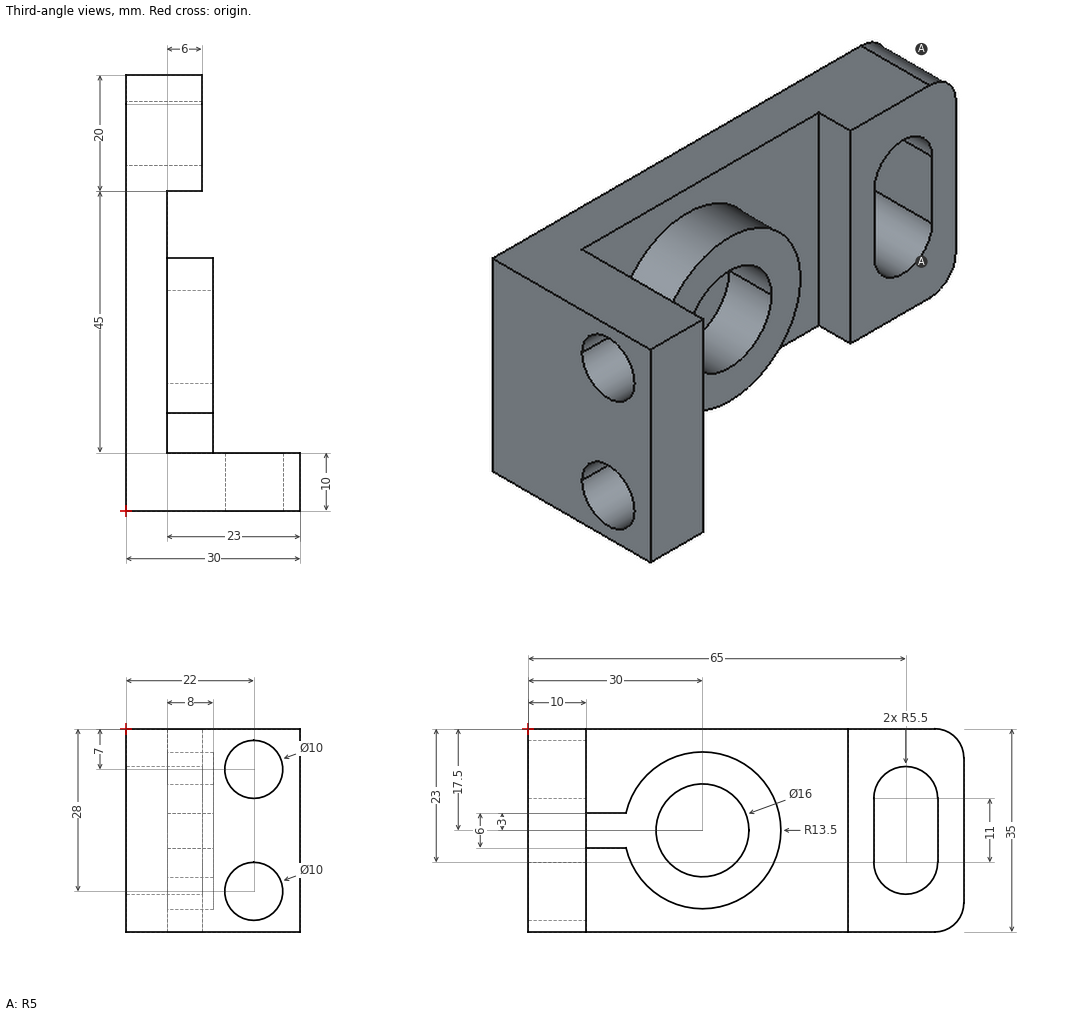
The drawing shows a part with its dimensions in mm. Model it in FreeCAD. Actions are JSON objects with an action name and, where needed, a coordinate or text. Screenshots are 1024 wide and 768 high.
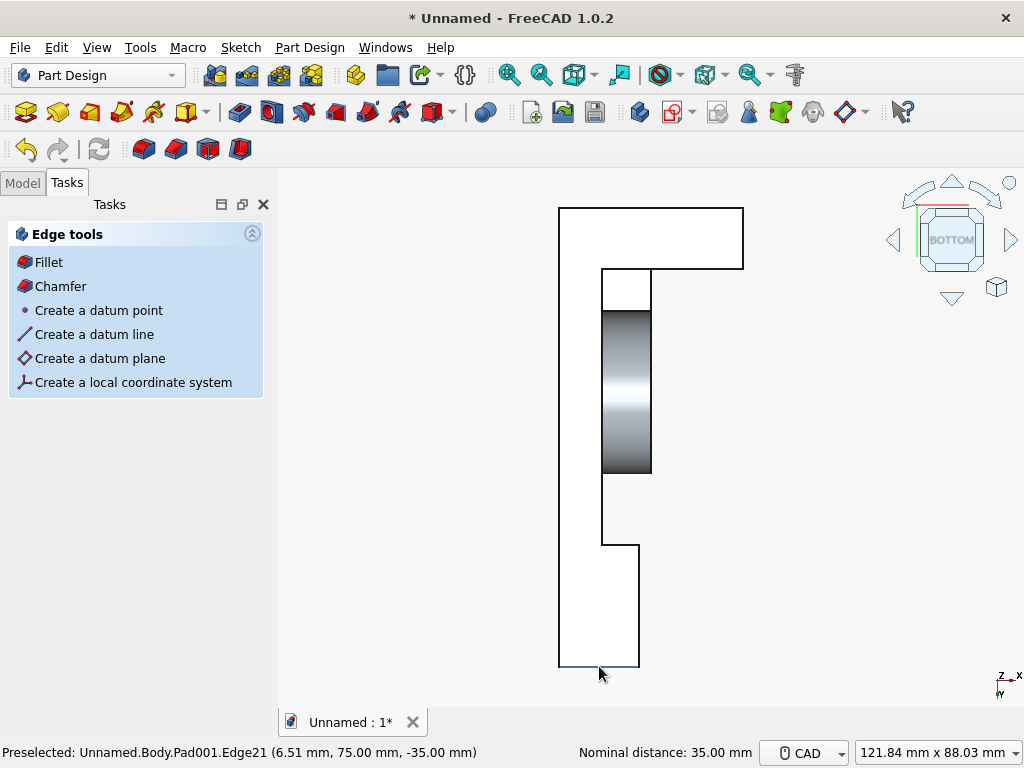
{"action": "left_click", "coordinate": [144, 150]}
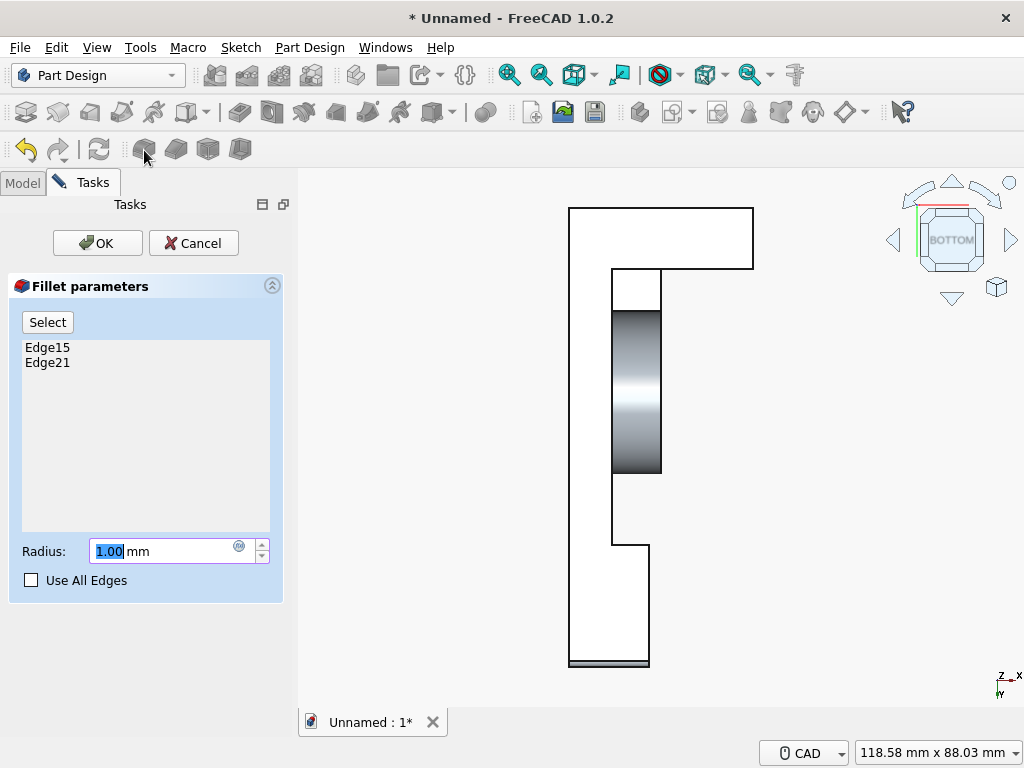
{"action": "type", "text": "5"}
{"action": "key", "text": "Tab"}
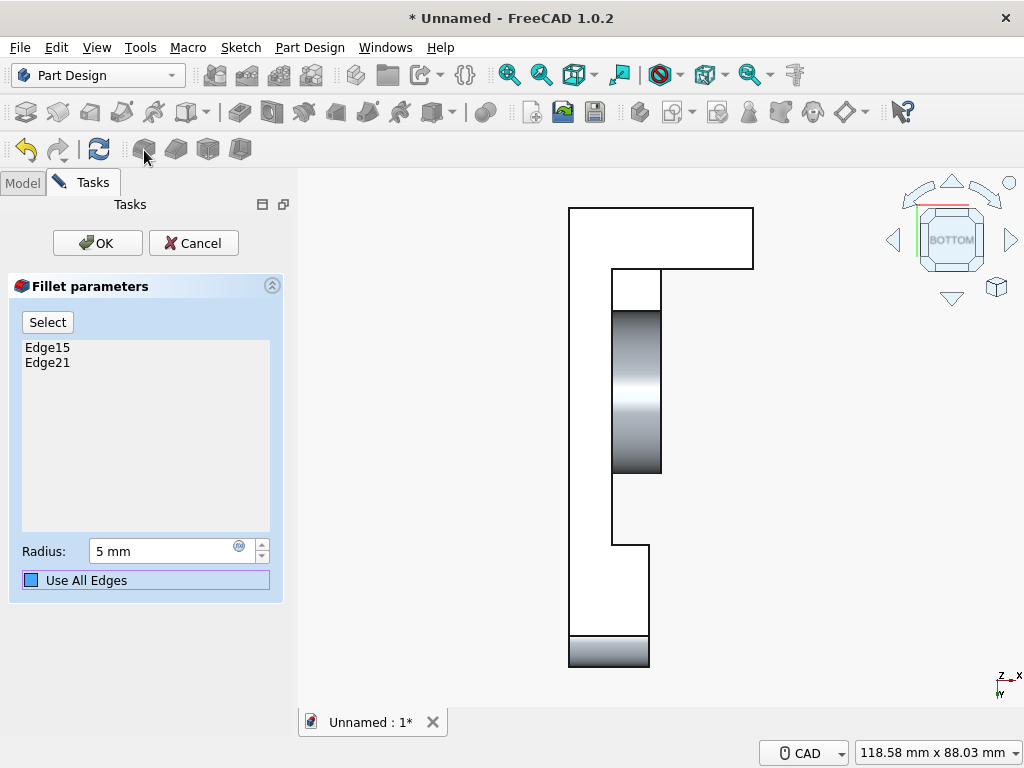
{"action": "left_click", "coordinate": [98, 243]}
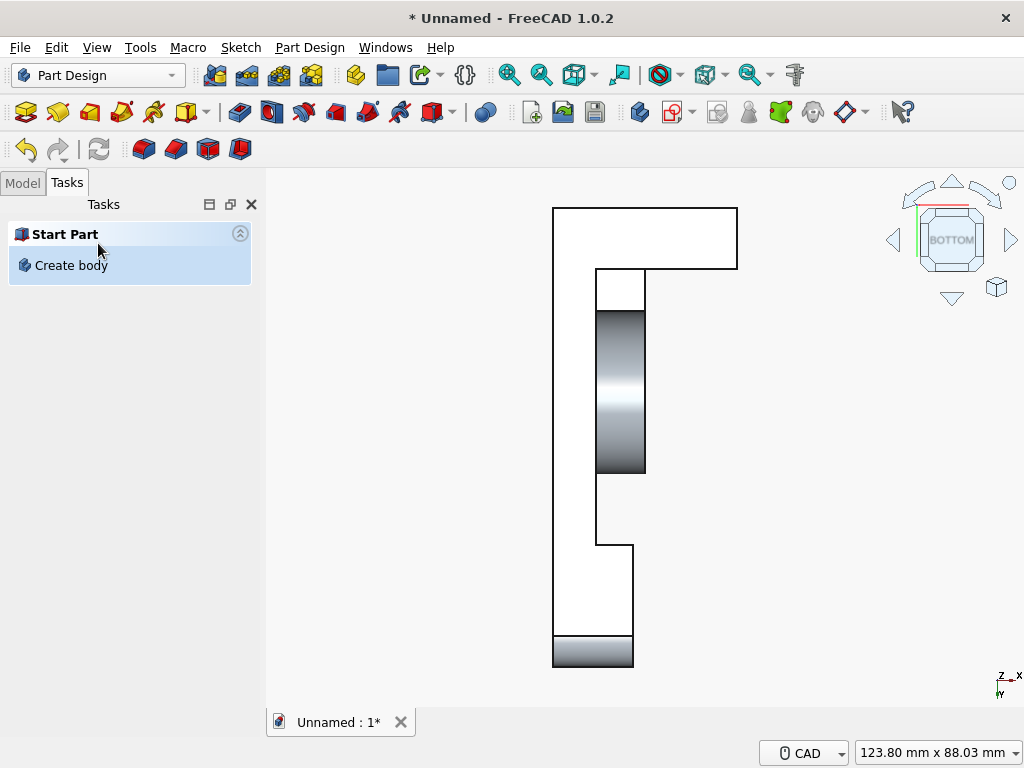
{"action": "key", "text": "0"}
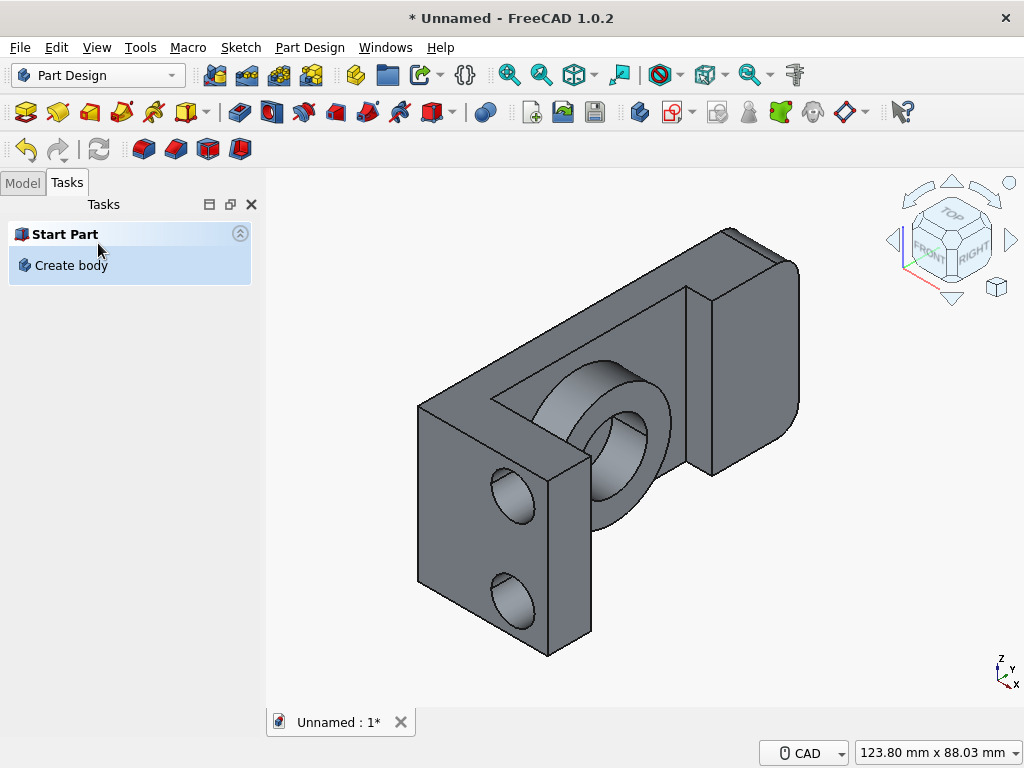
{"action": "left_click", "coordinate": [755, 338]}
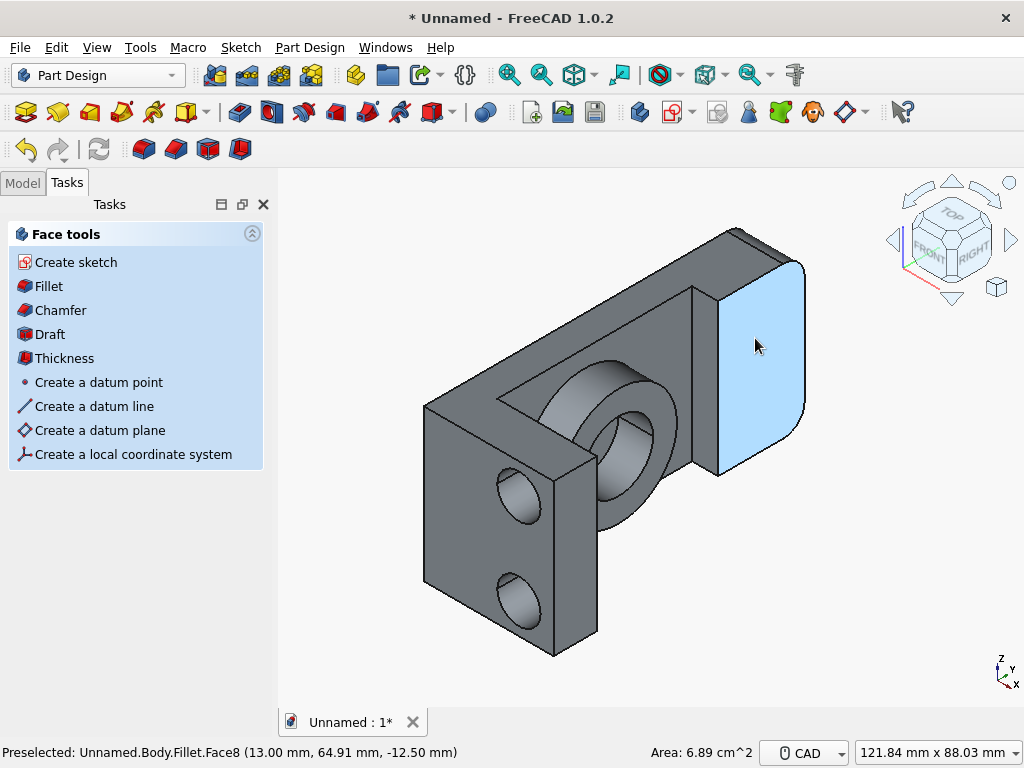
{"action": "left_click", "coordinate": [672, 112]}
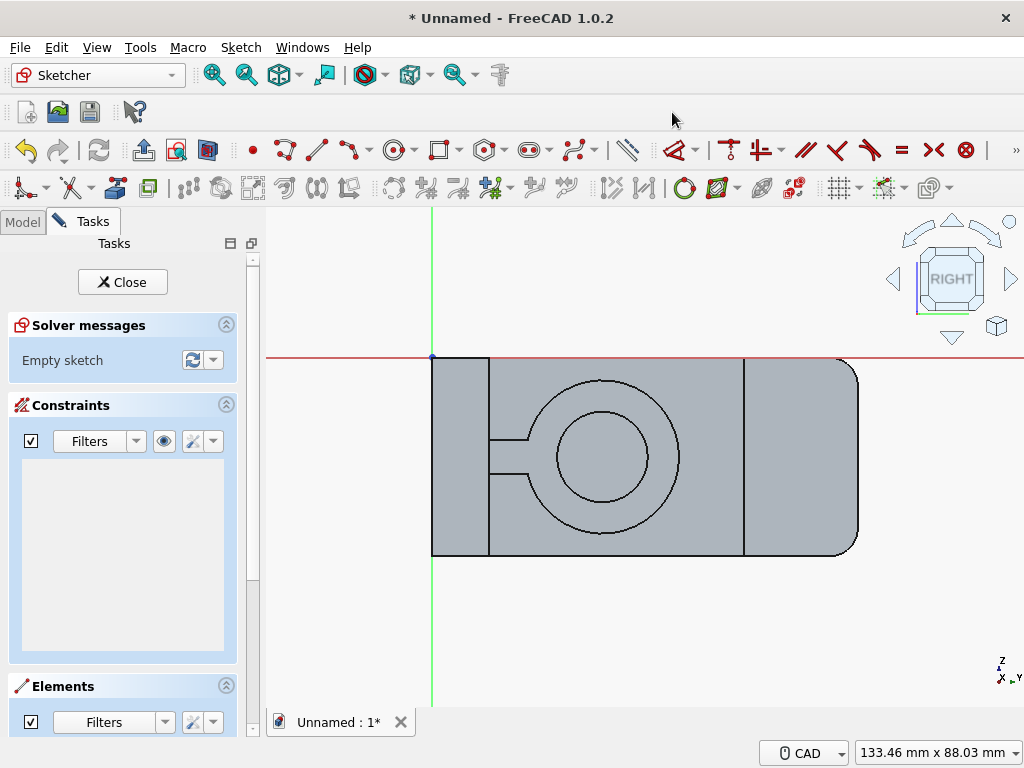
{"action": "scroll", "coordinate": [859, 457], "scroll_direction": "up", "scroll_amount": 5}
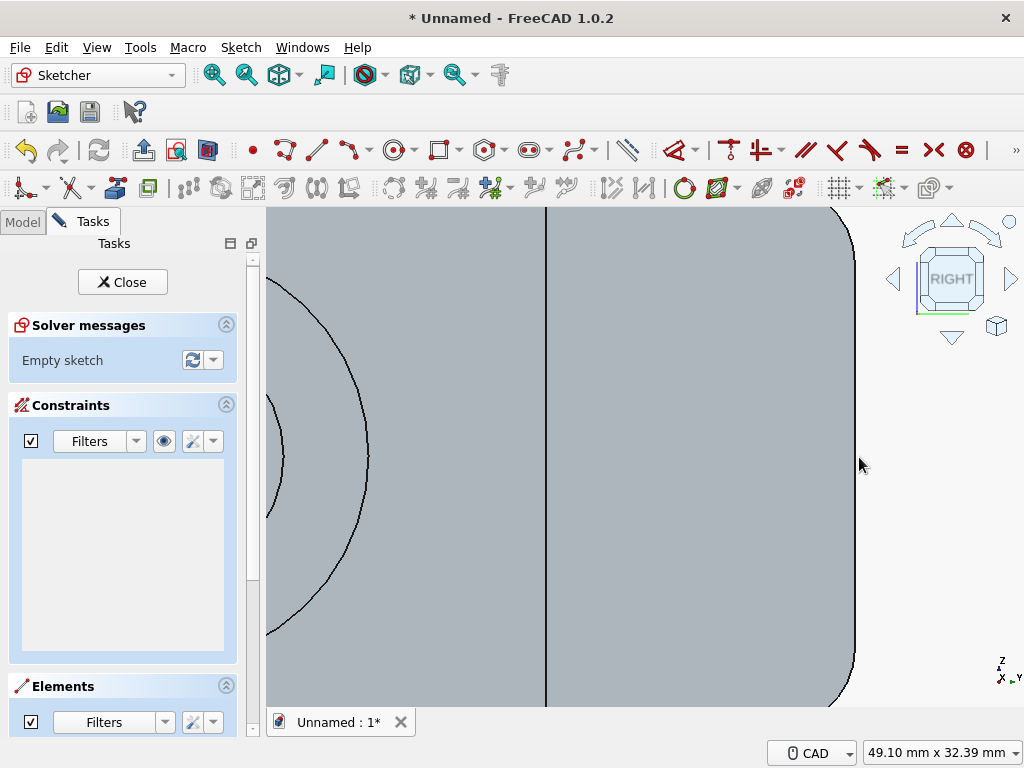
{"action": "left_click", "coordinate": [530, 150]}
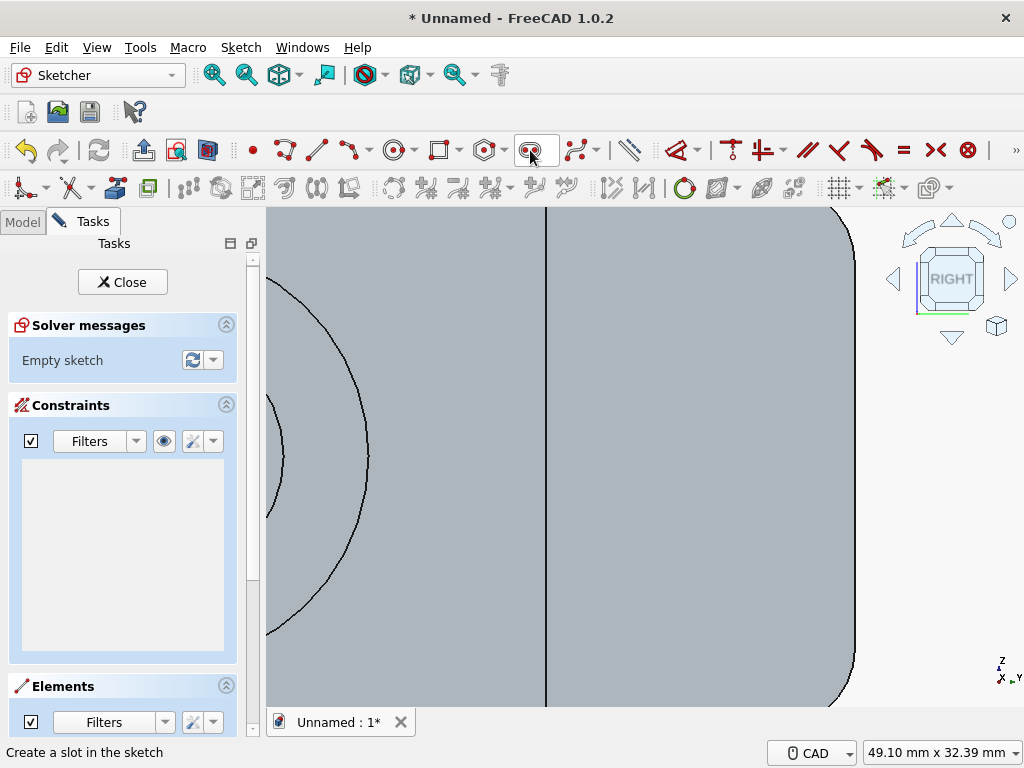
{"action": "left_click", "coordinate": [701, 541]}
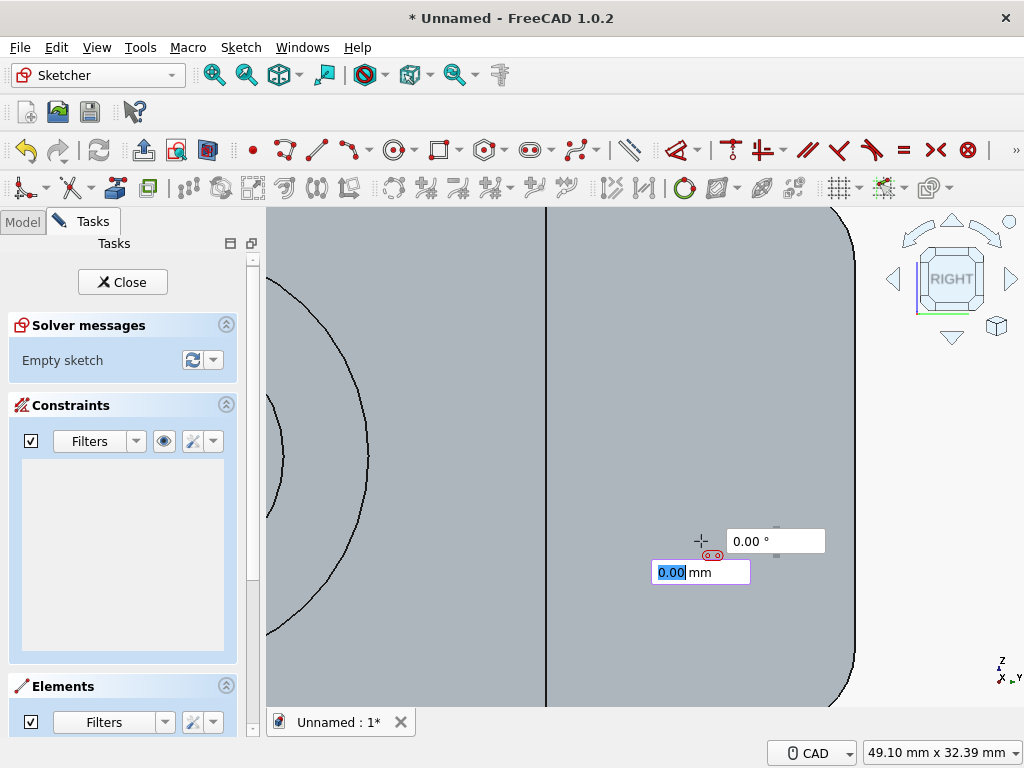
{"action": "left_click", "coordinate": [701, 371]}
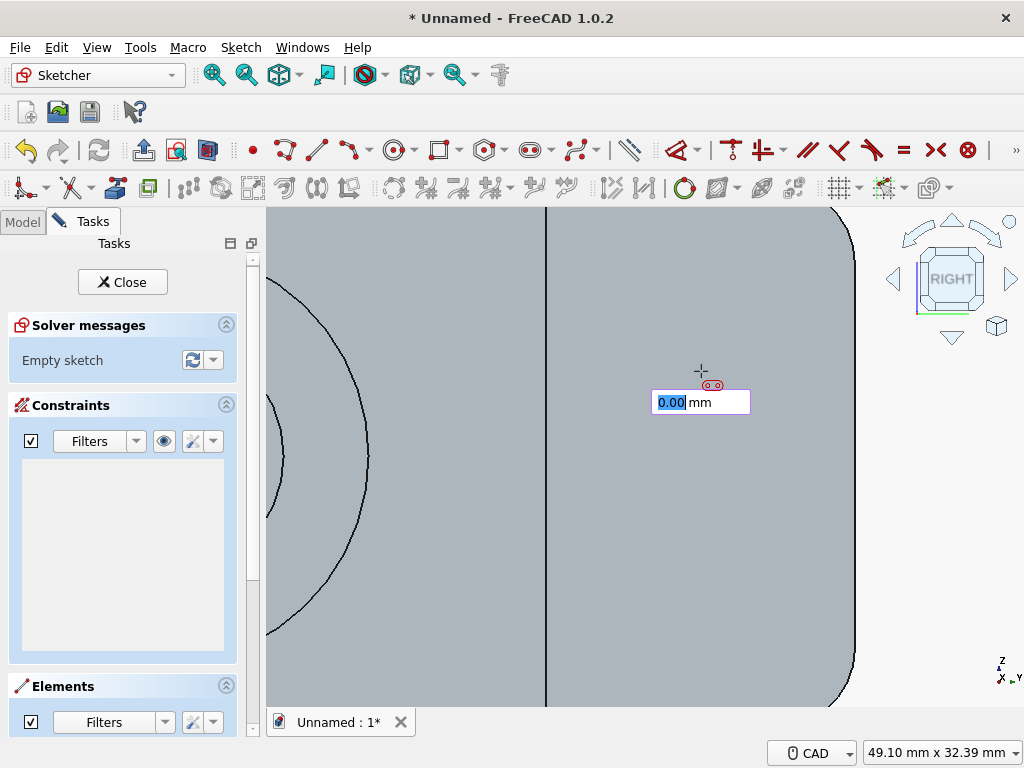
{"action": "left_click", "coordinate": [785, 456]}
{"action": "key", "text": "Escape"}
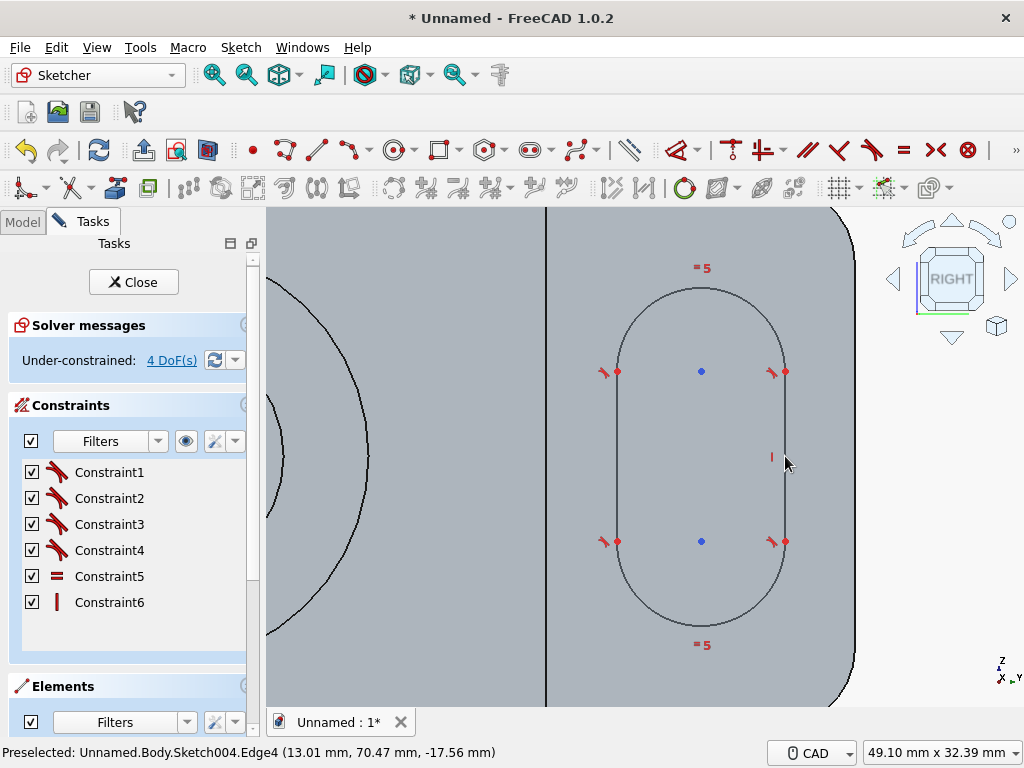
{"action": "left_click", "coordinate": [676, 150]}